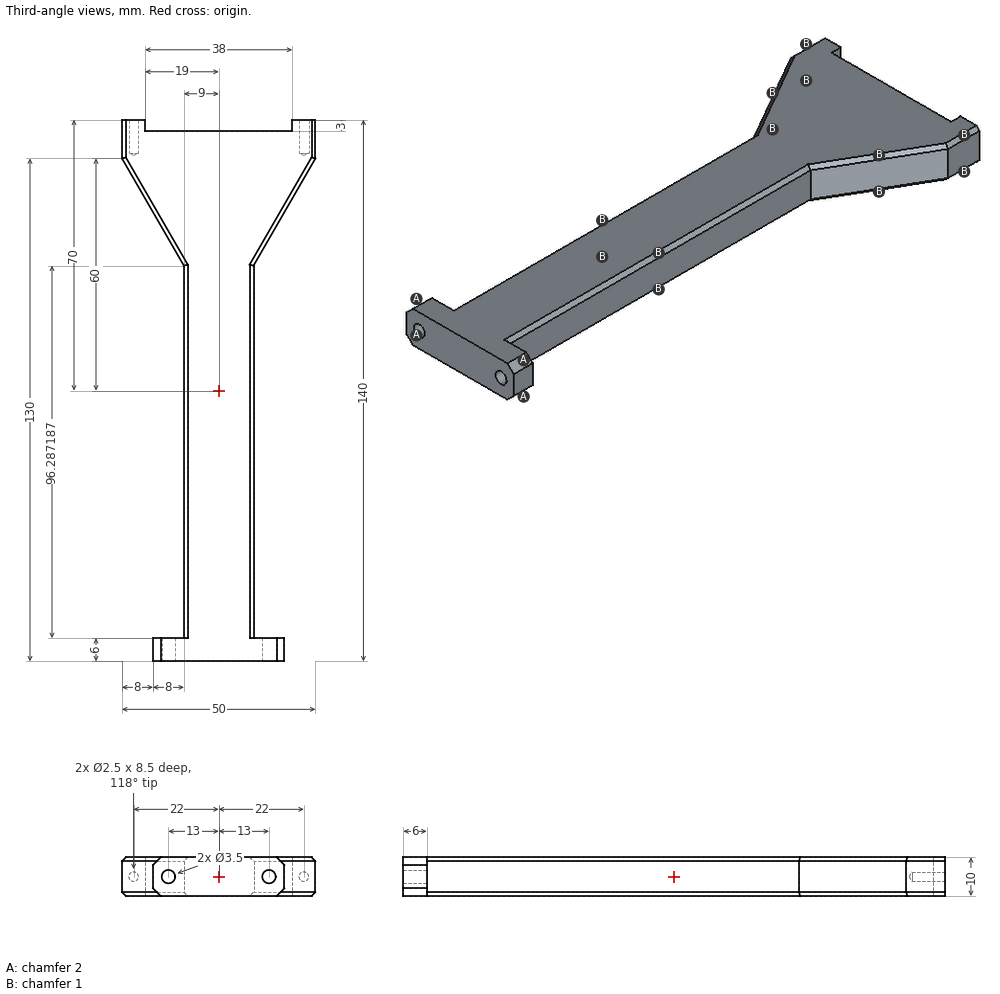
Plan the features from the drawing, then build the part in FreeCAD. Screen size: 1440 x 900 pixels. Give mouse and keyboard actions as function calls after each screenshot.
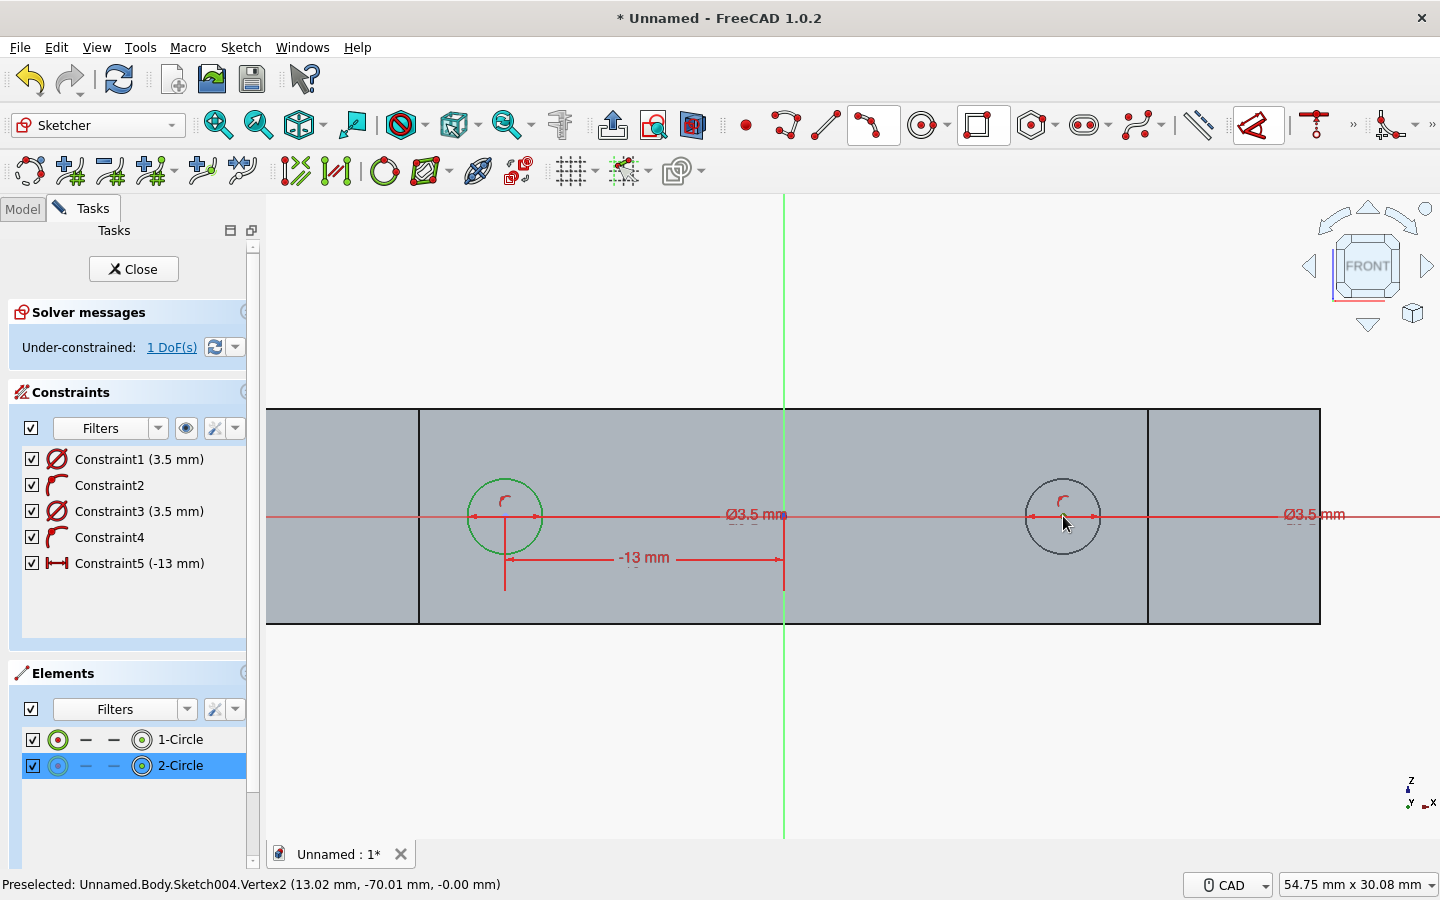
click(1278, 126)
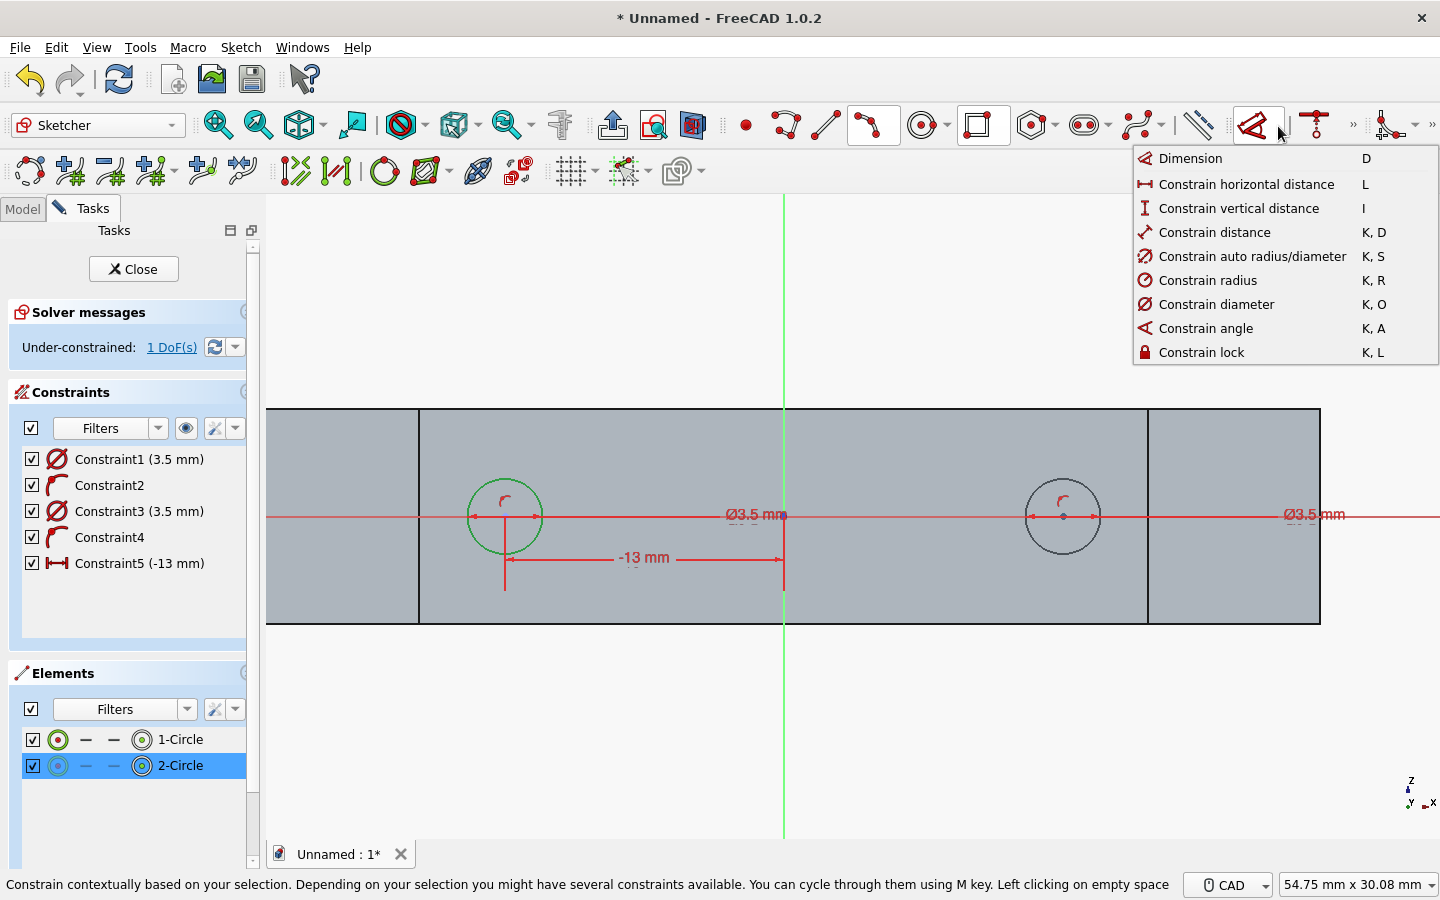
click(1286, 184)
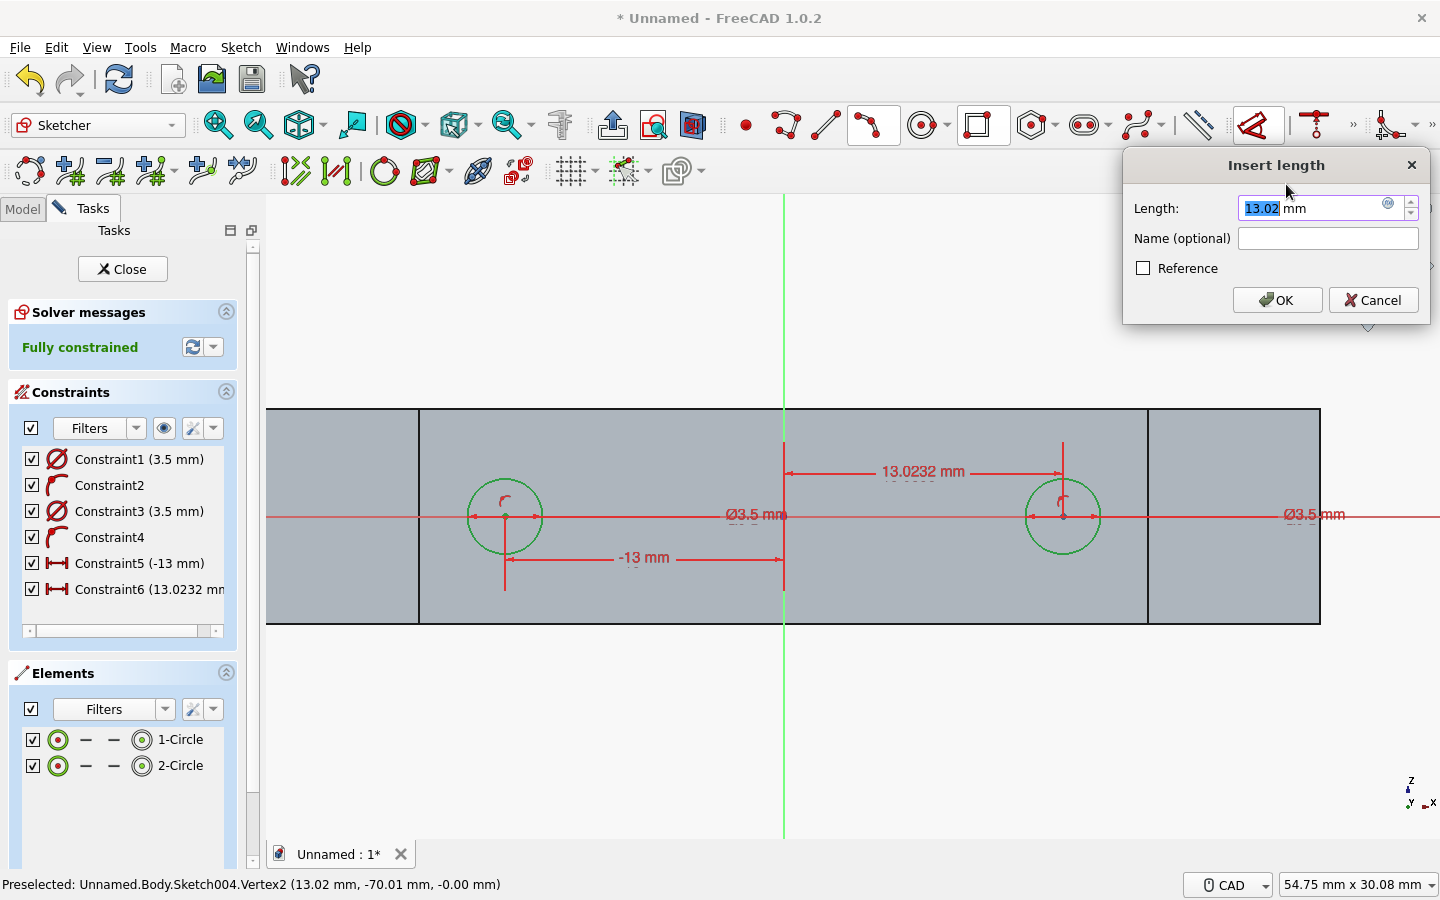
text(13)
key(Return)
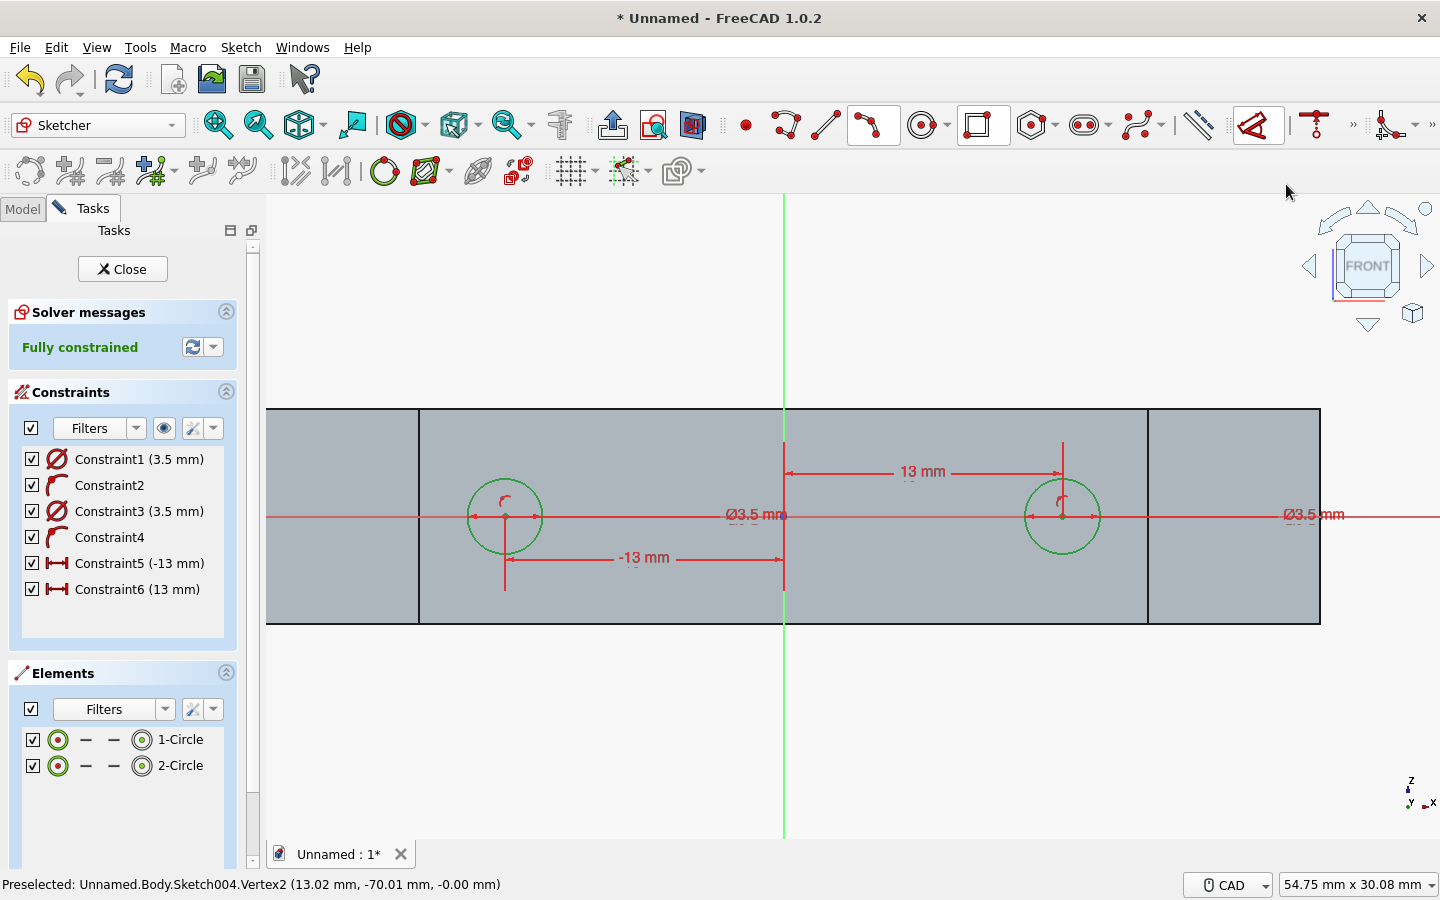
click(123, 269)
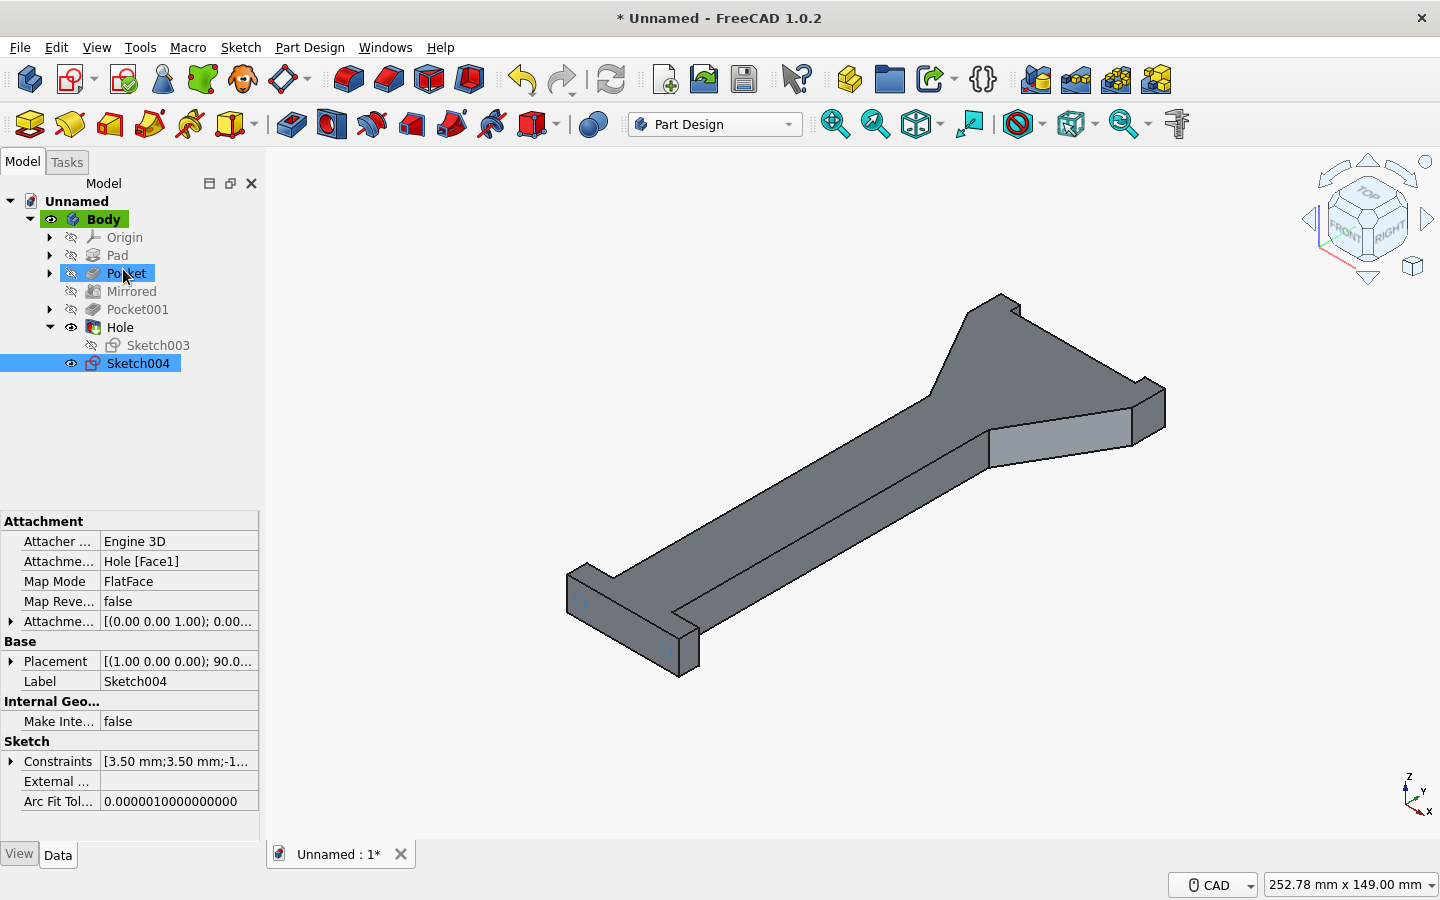
click(292, 124)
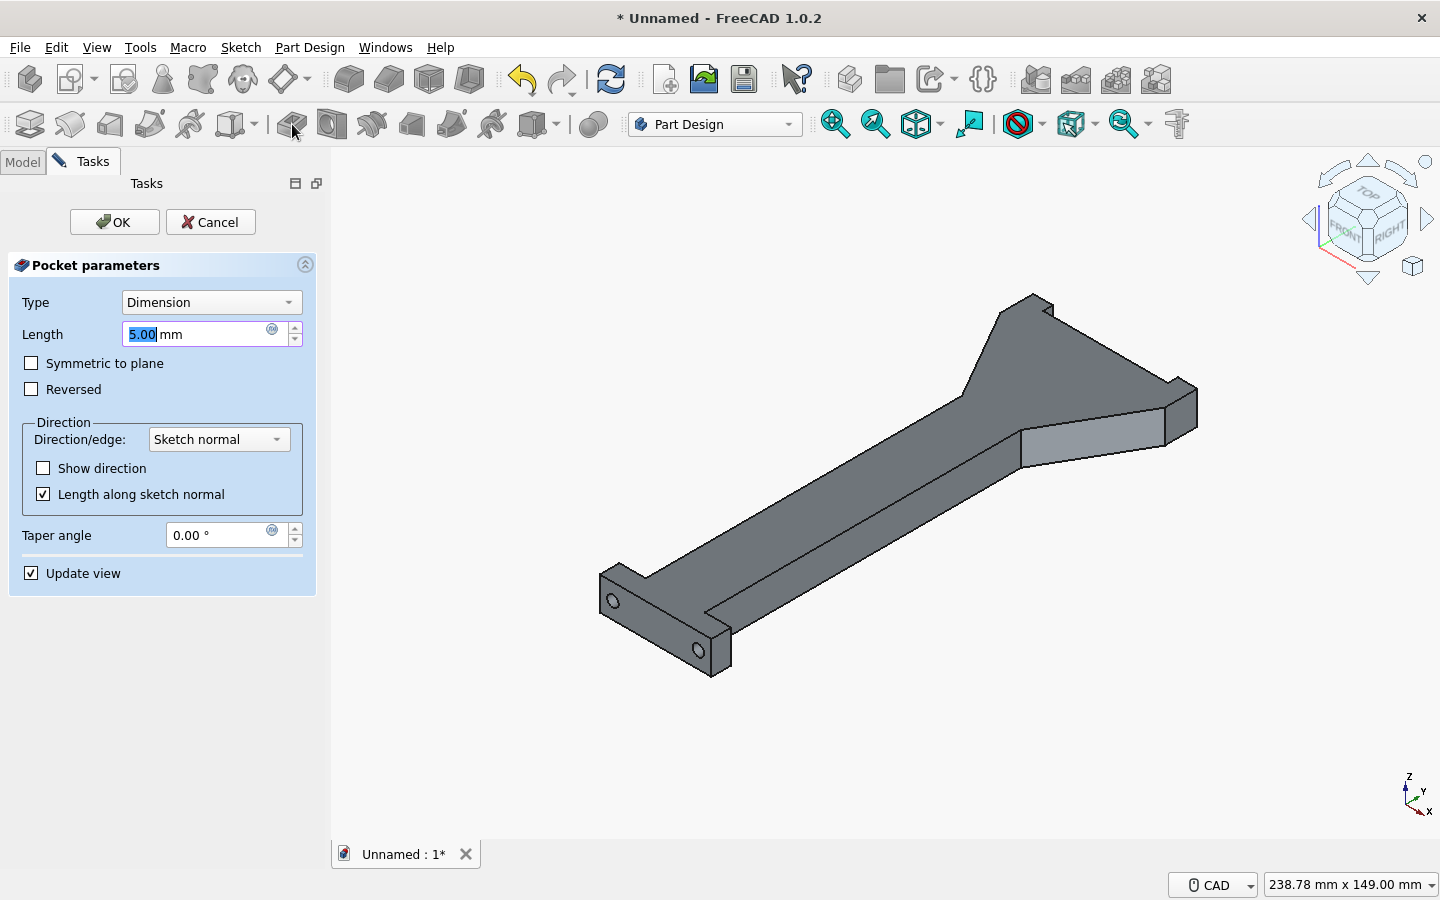
text(6)
key(Tab)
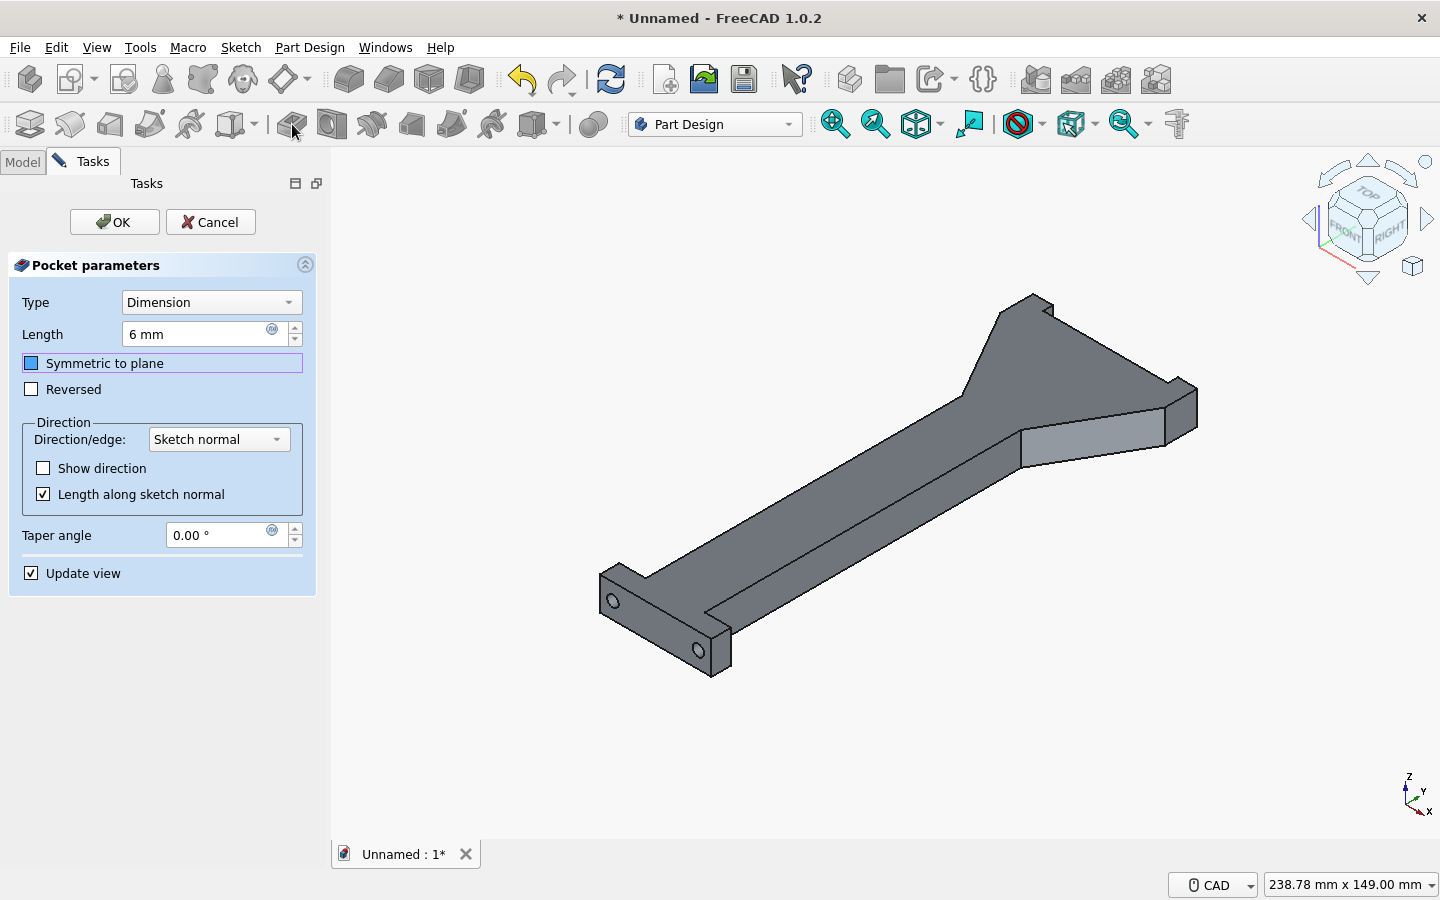
click(115, 222)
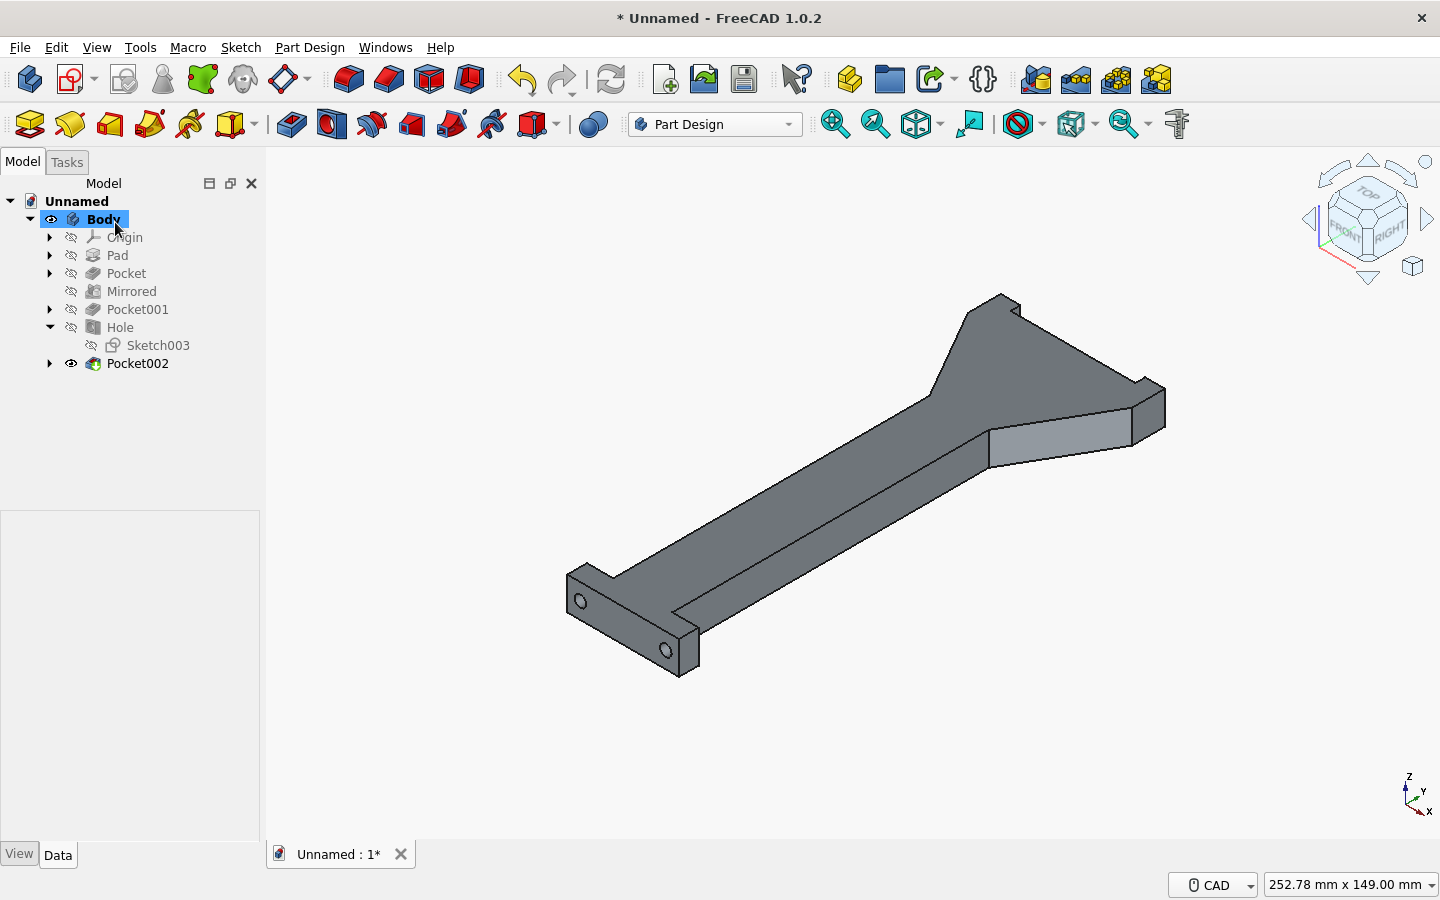
click(689, 632)